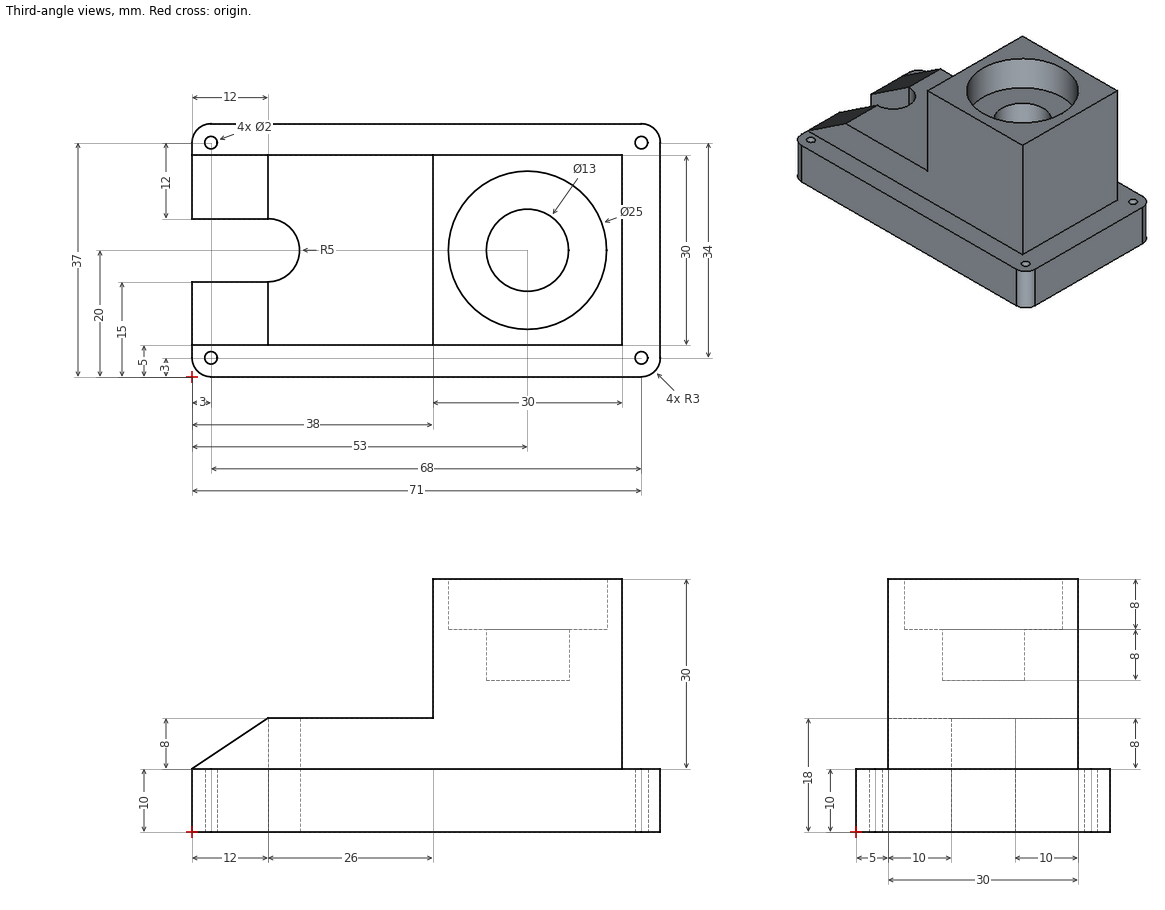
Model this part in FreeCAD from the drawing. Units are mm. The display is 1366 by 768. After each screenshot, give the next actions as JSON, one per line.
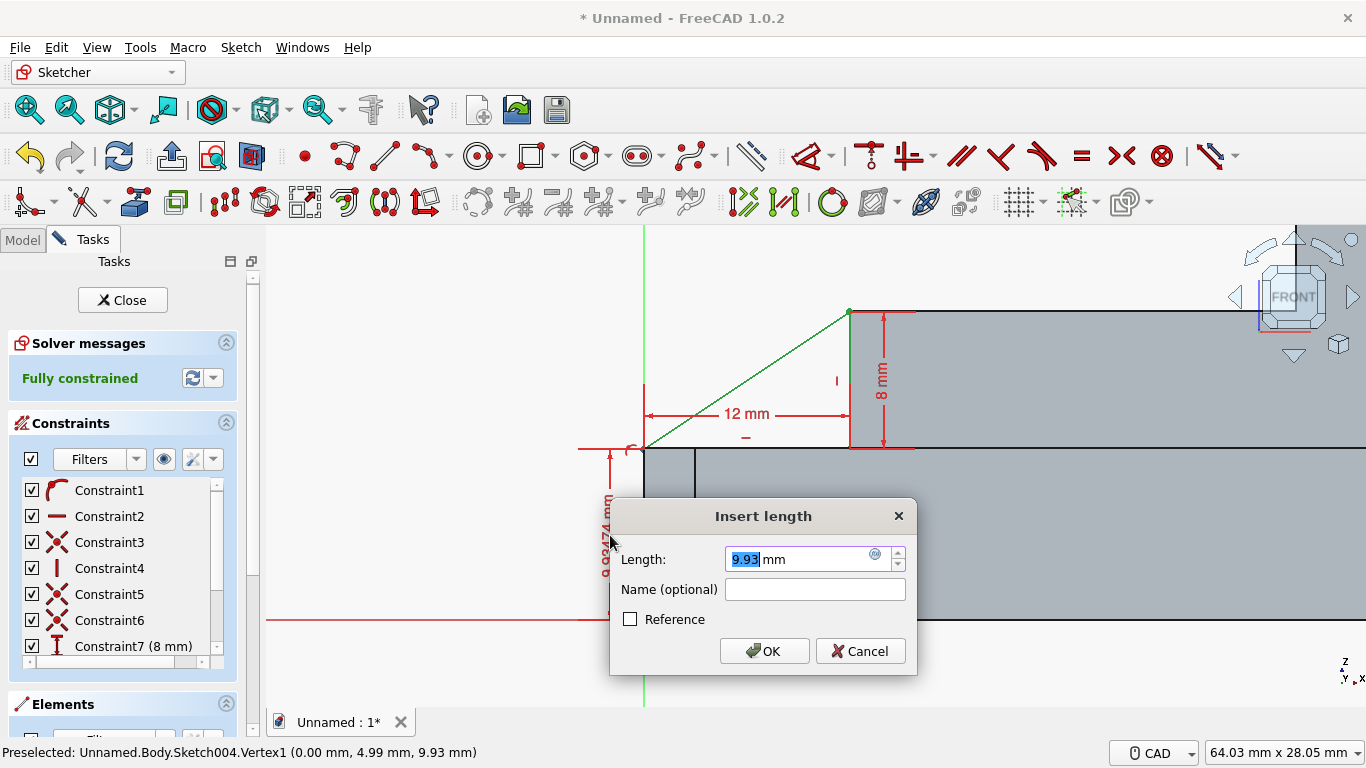
{"action": "type", "text": "10"}
{"action": "key", "text": "Return"}
{"action": "key", "text": "Escape"}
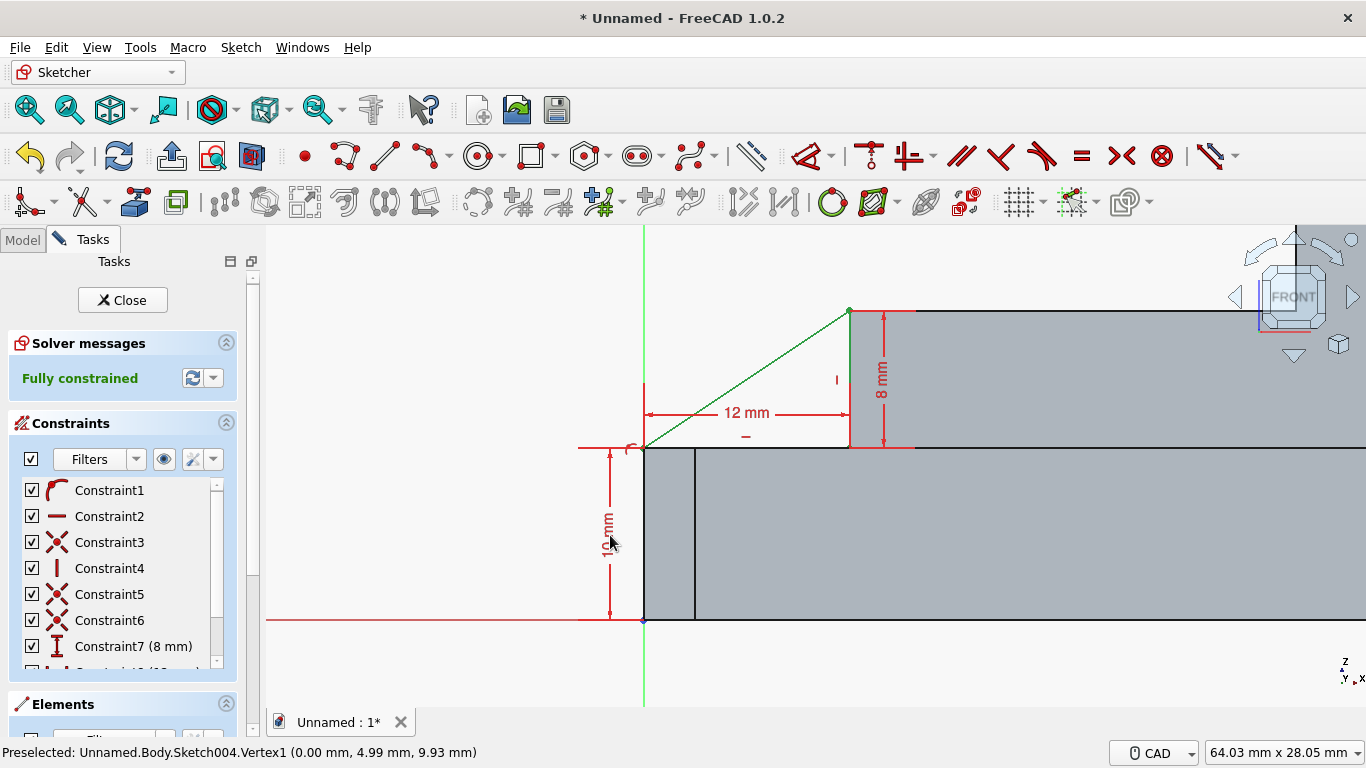
{"action": "left_click", "coordinate": [123, 300]}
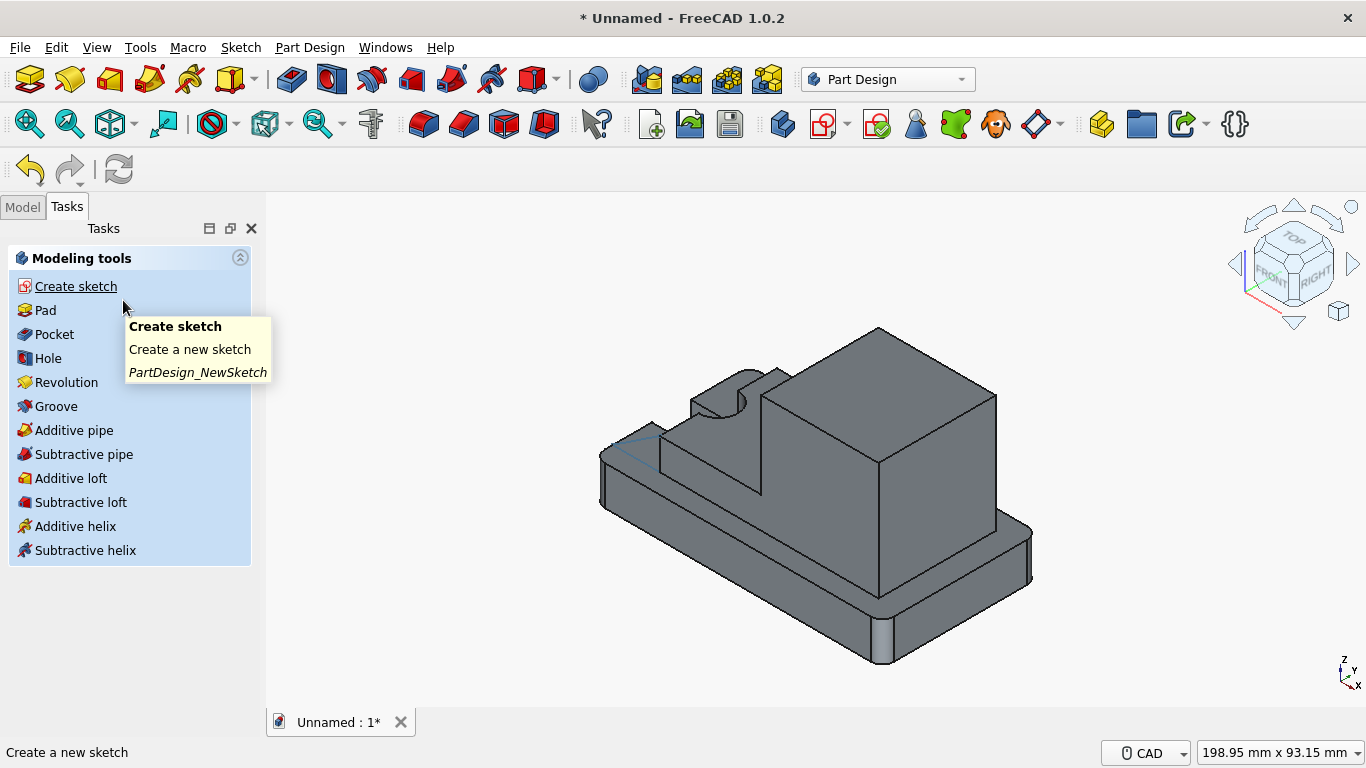
{"action": "left_click", "coordinate": [30, 80]}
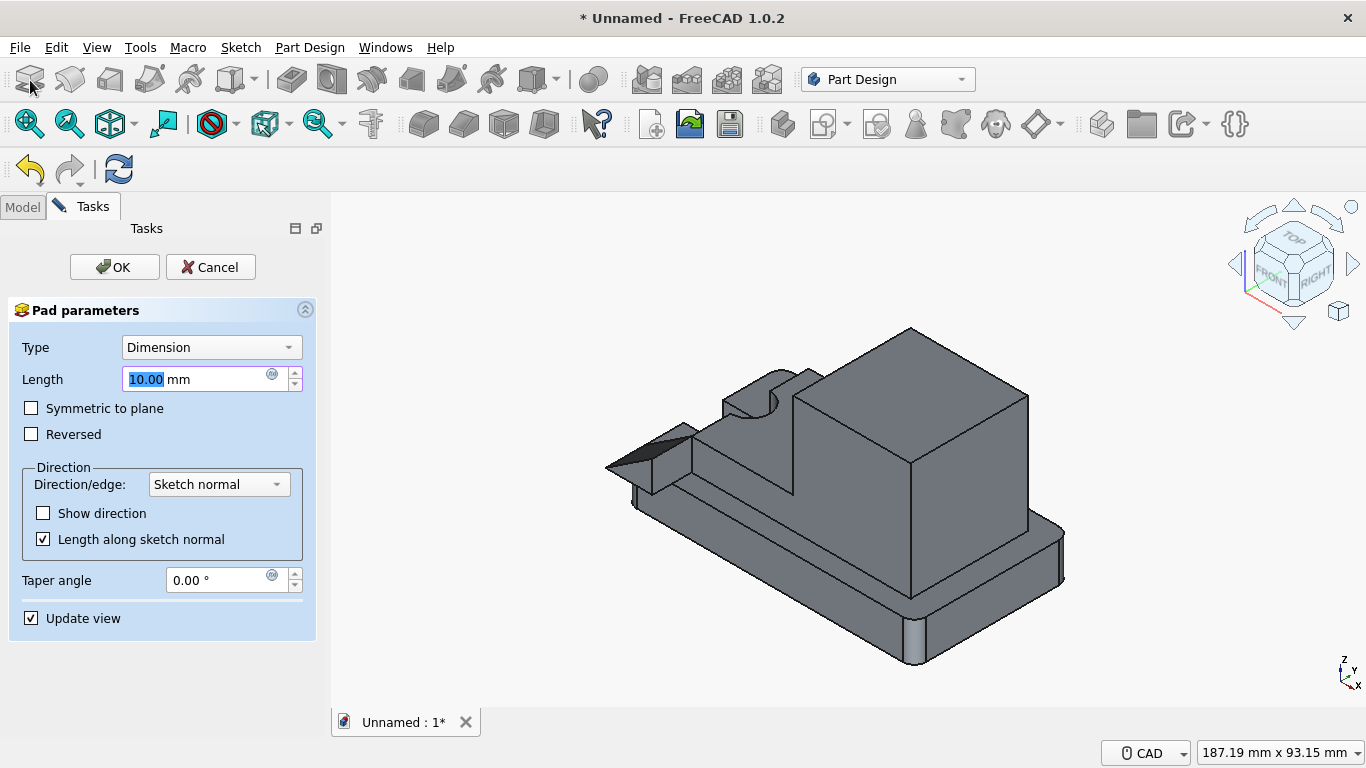
{"action": "type", "text": "10"}
{"action": "key", "text": "Tab"}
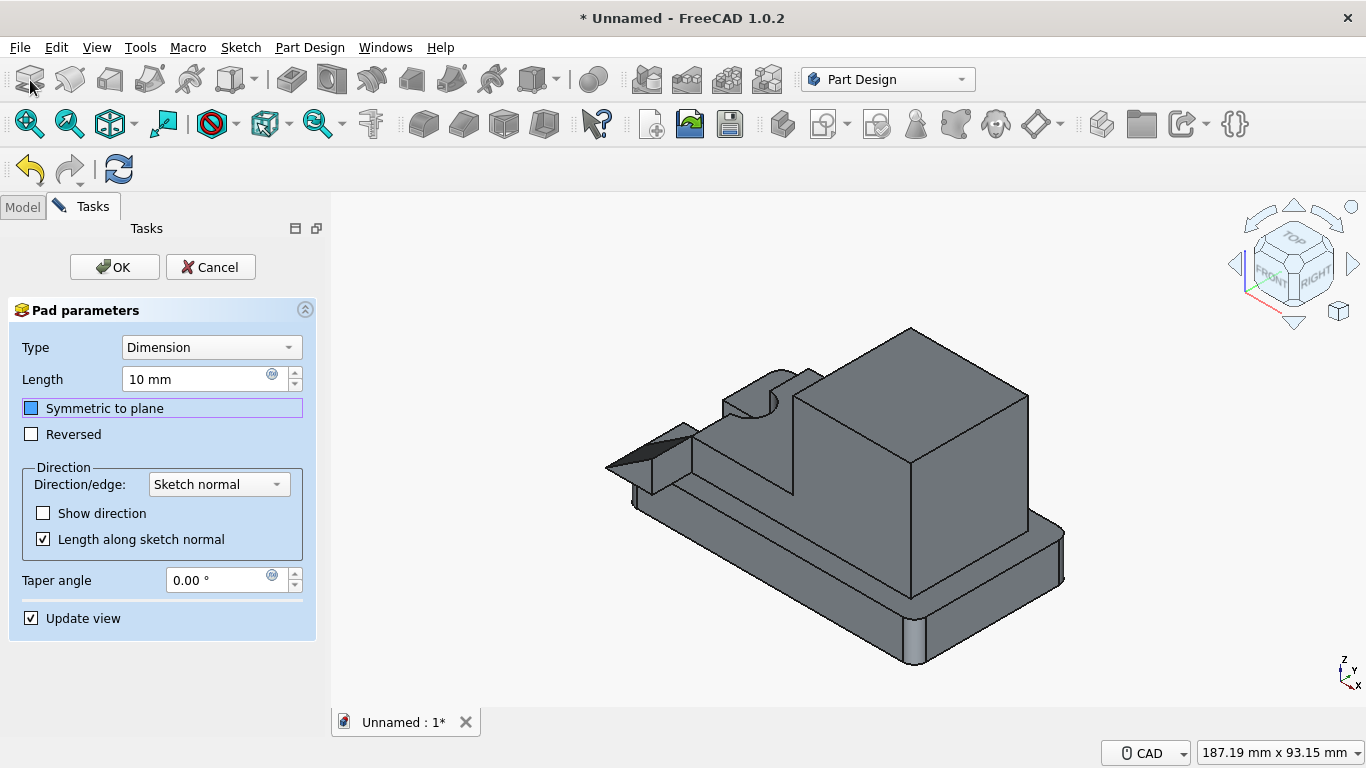
{"action": "left_click", "coordinate": [30, 434]}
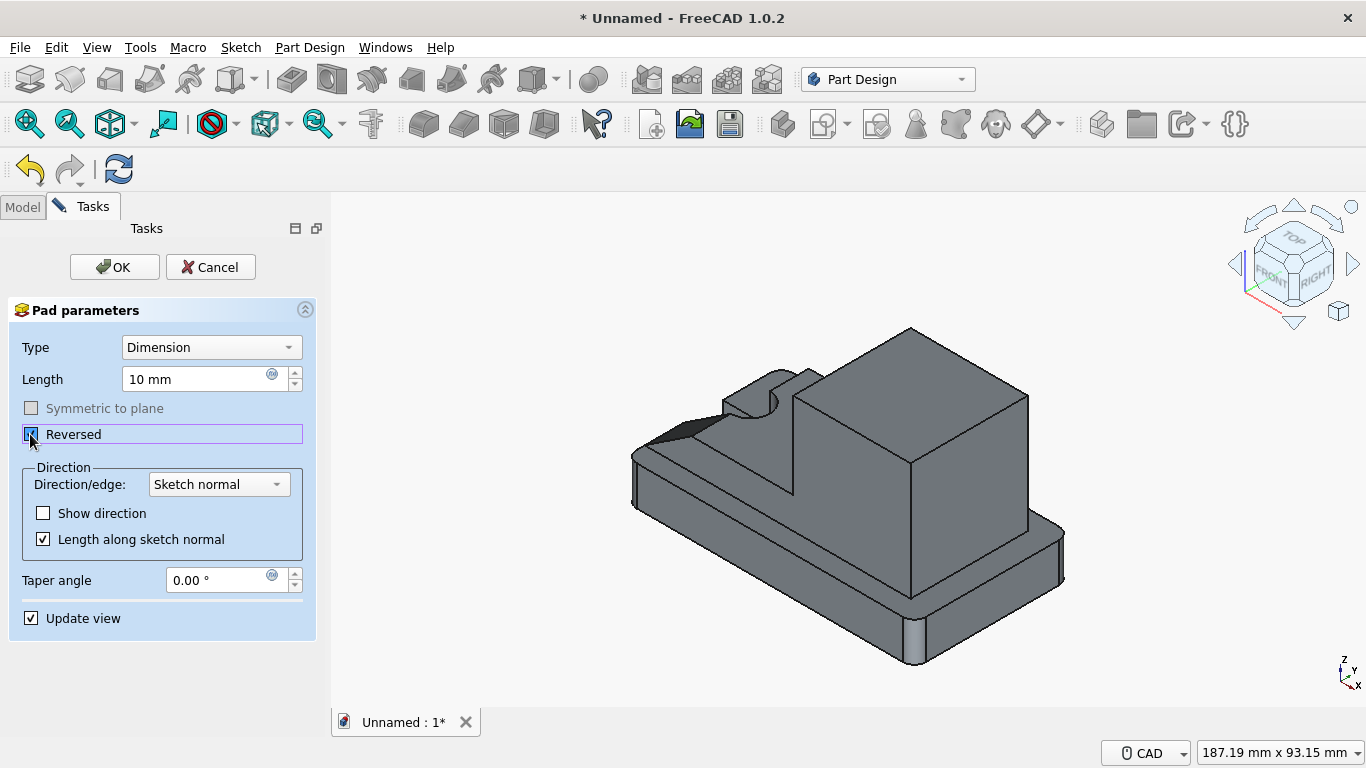
{"action": "left_click", "coordinate": [115, 267]}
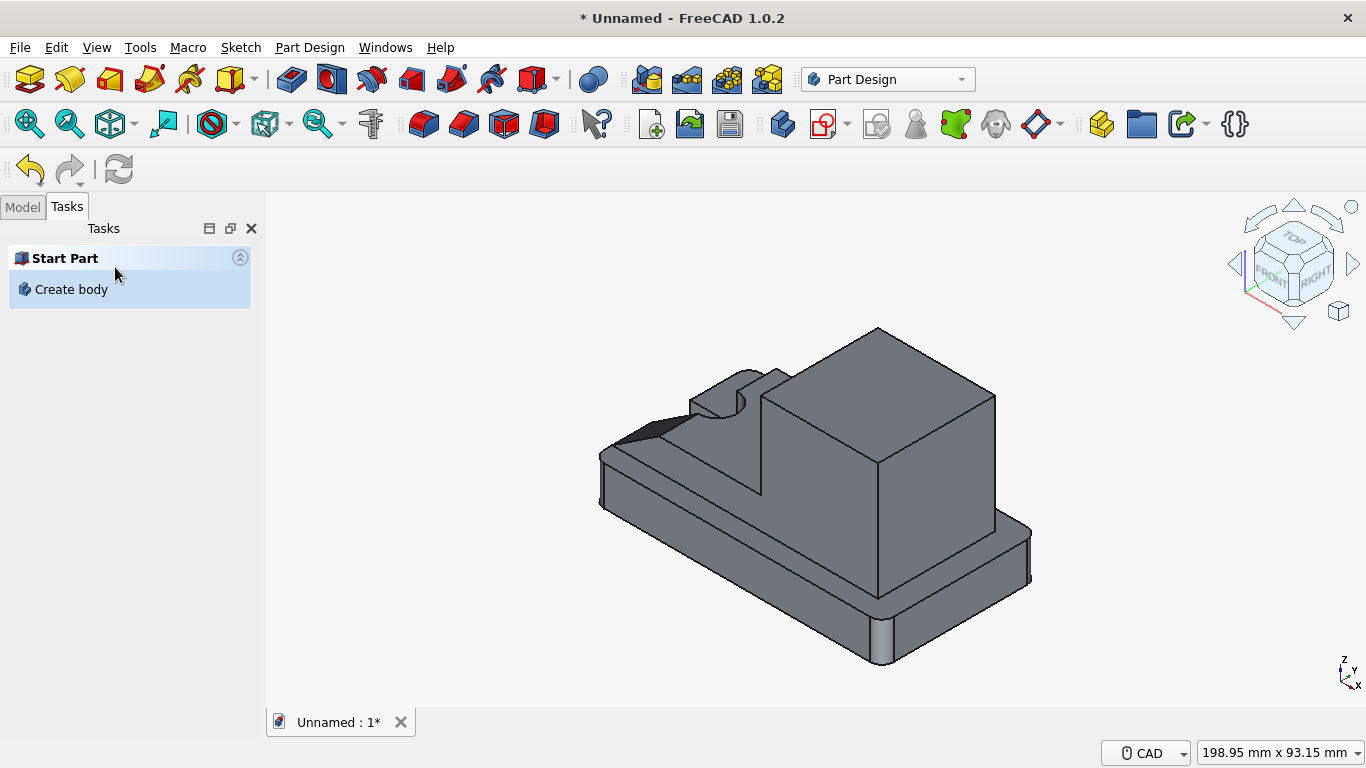
{"action": "key", "text": "4"}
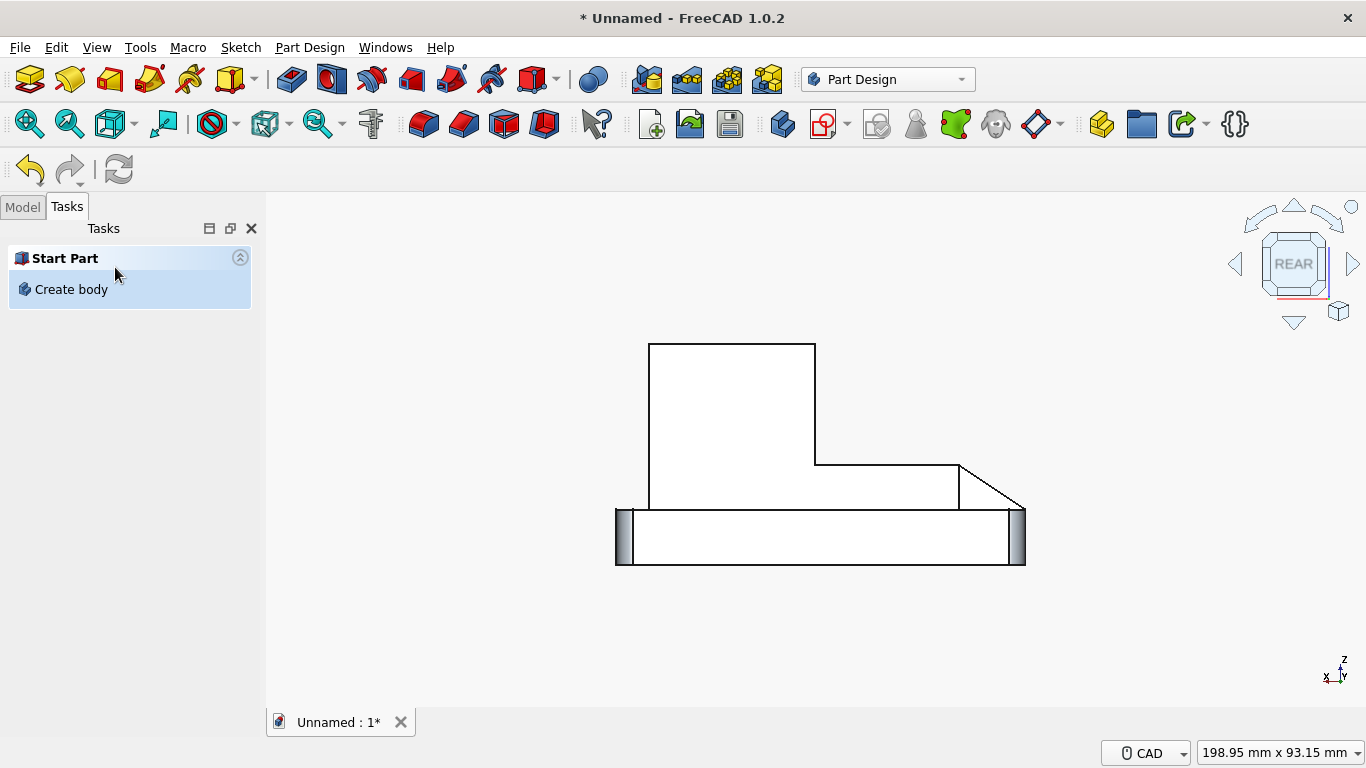
{"action": "left_click", "coordinate": [30, 124]}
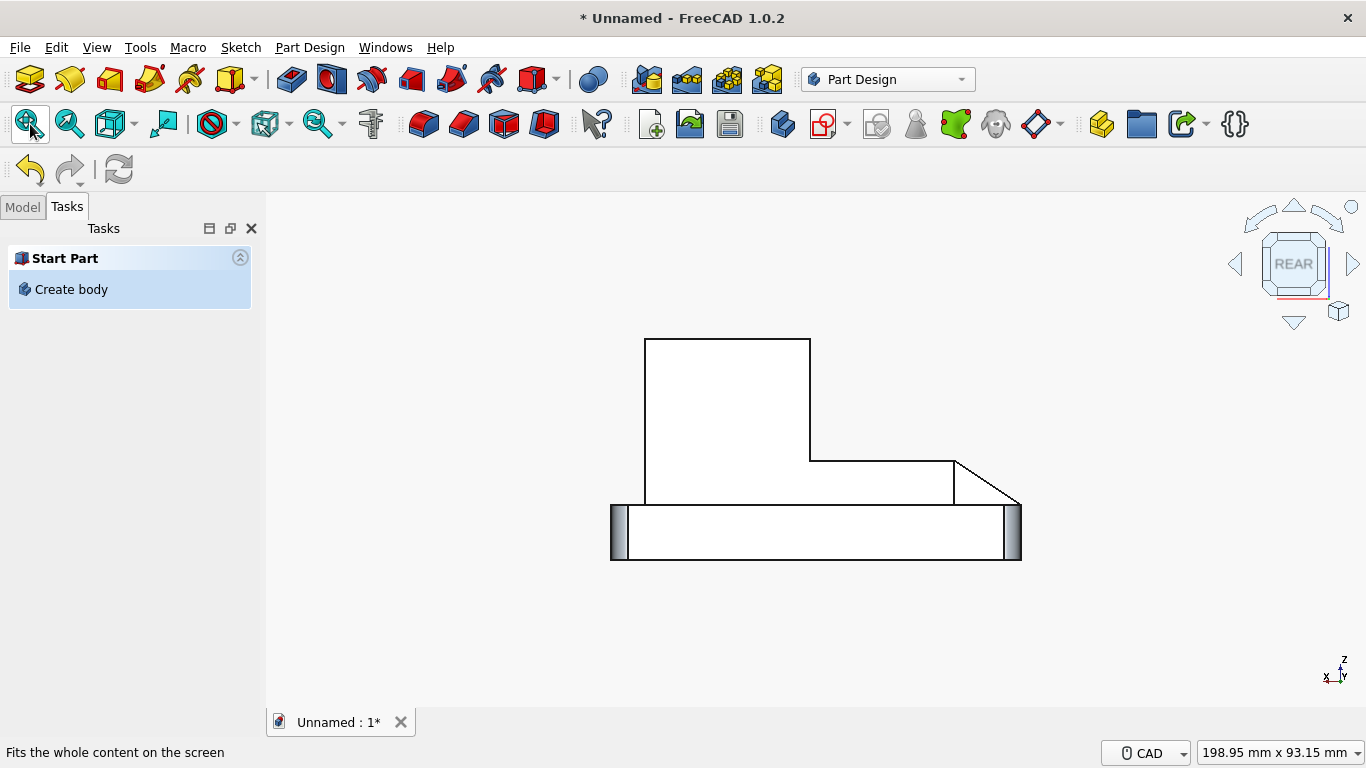
{"action": "left_click", "coordinate": [711, 421]}